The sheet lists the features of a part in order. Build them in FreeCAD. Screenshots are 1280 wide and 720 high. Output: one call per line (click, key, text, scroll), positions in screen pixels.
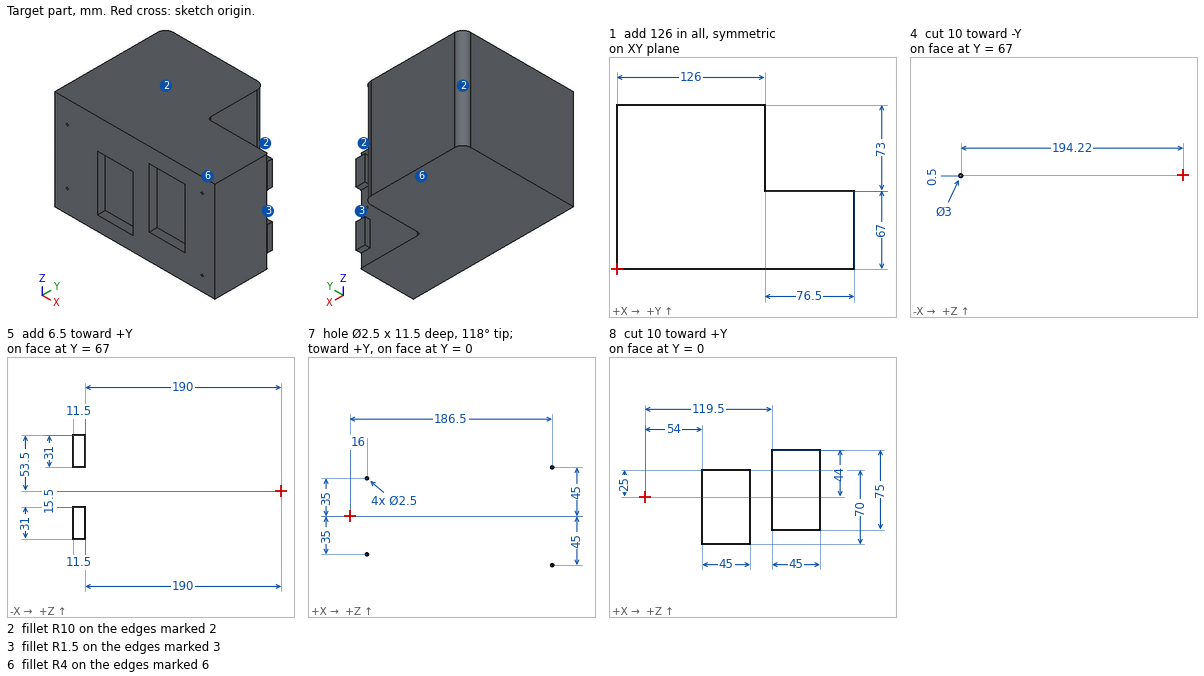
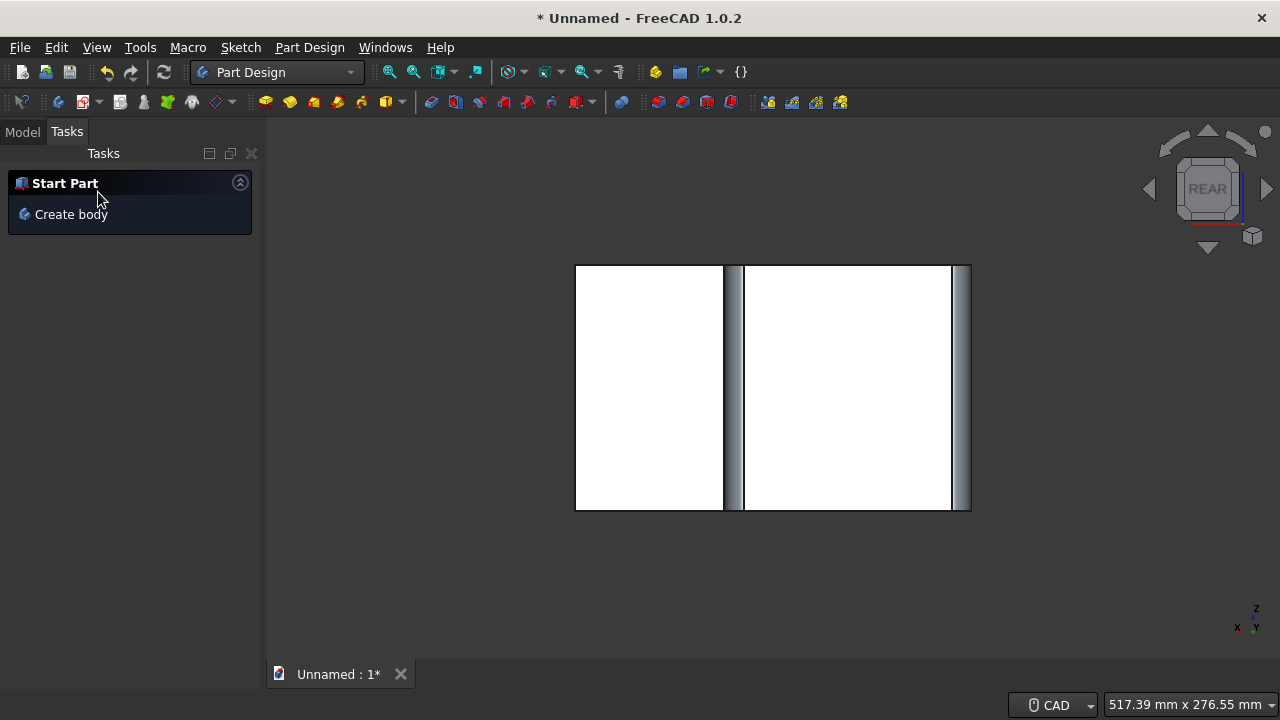
click(575, 387)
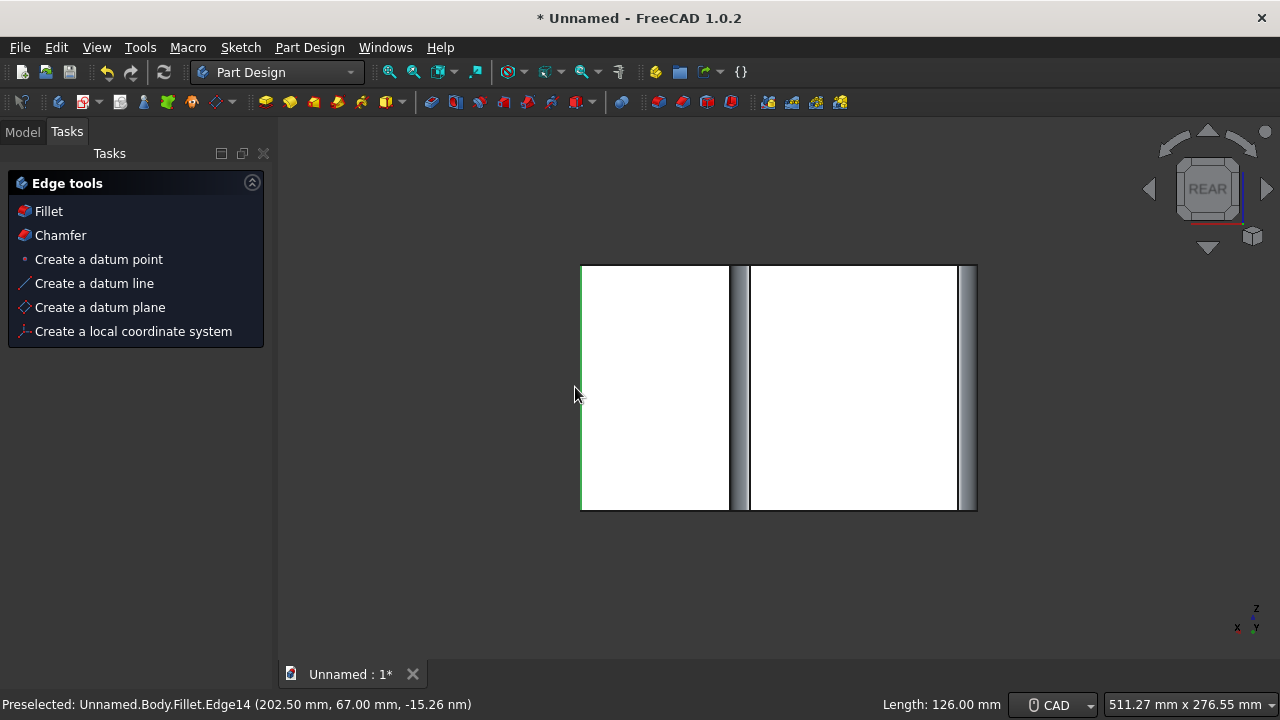
click(660, 102)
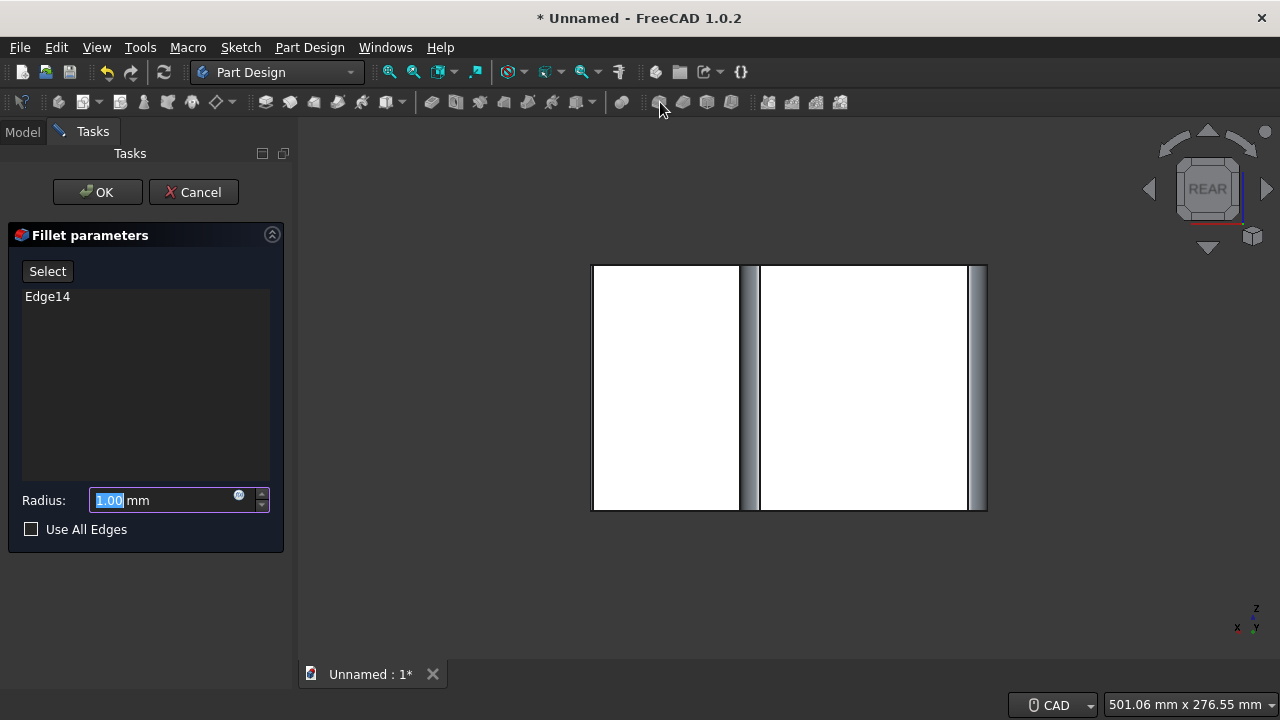
text(1.5)
key(Tab)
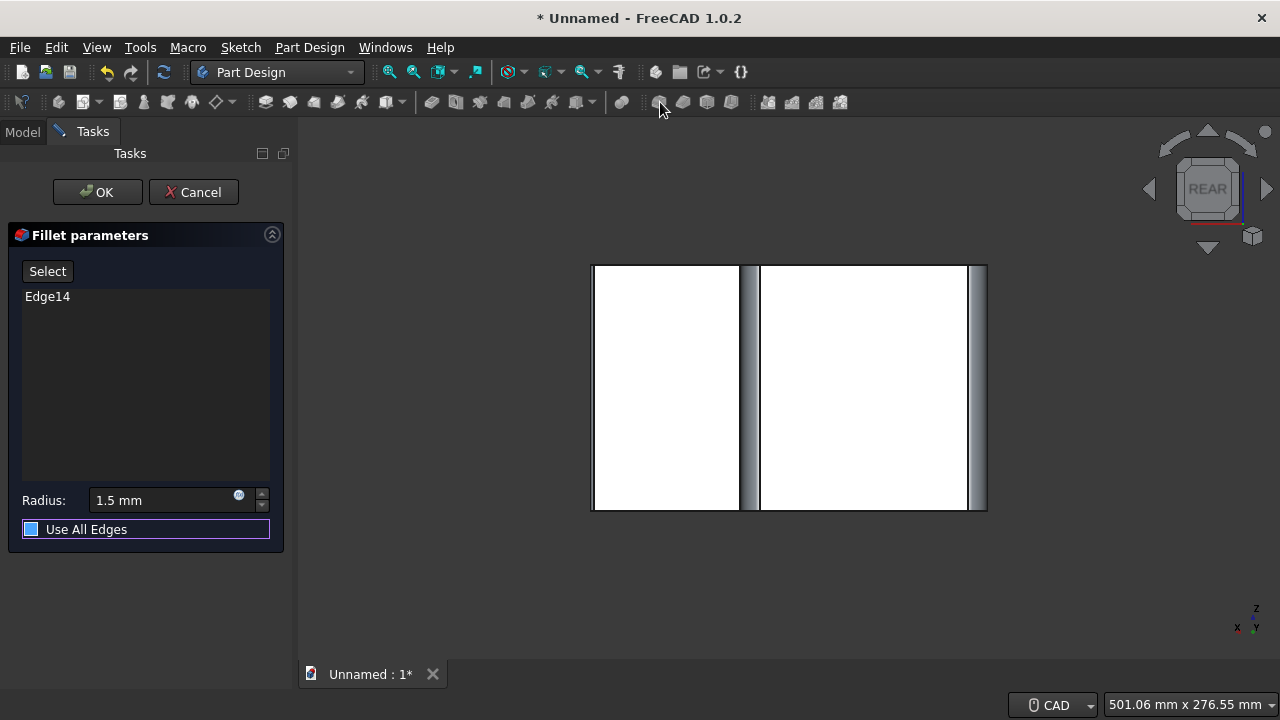
click(98, 192)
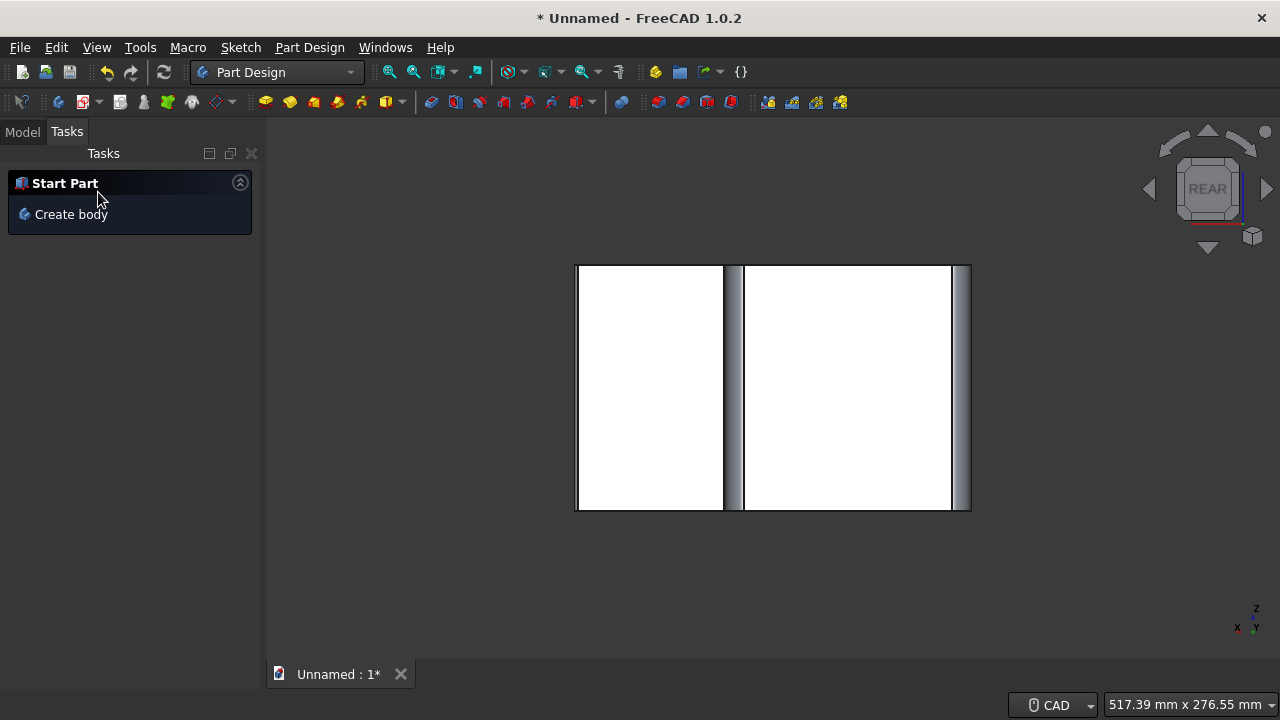
click(651, 352)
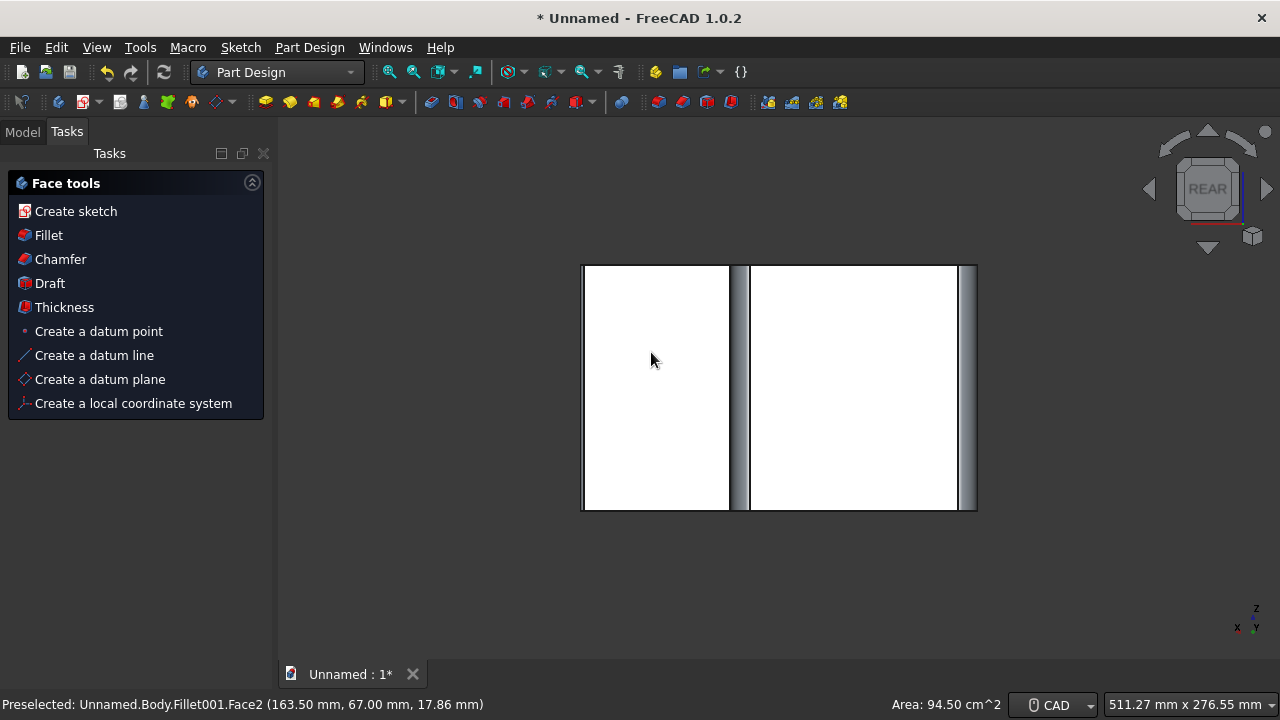
click(84, 102)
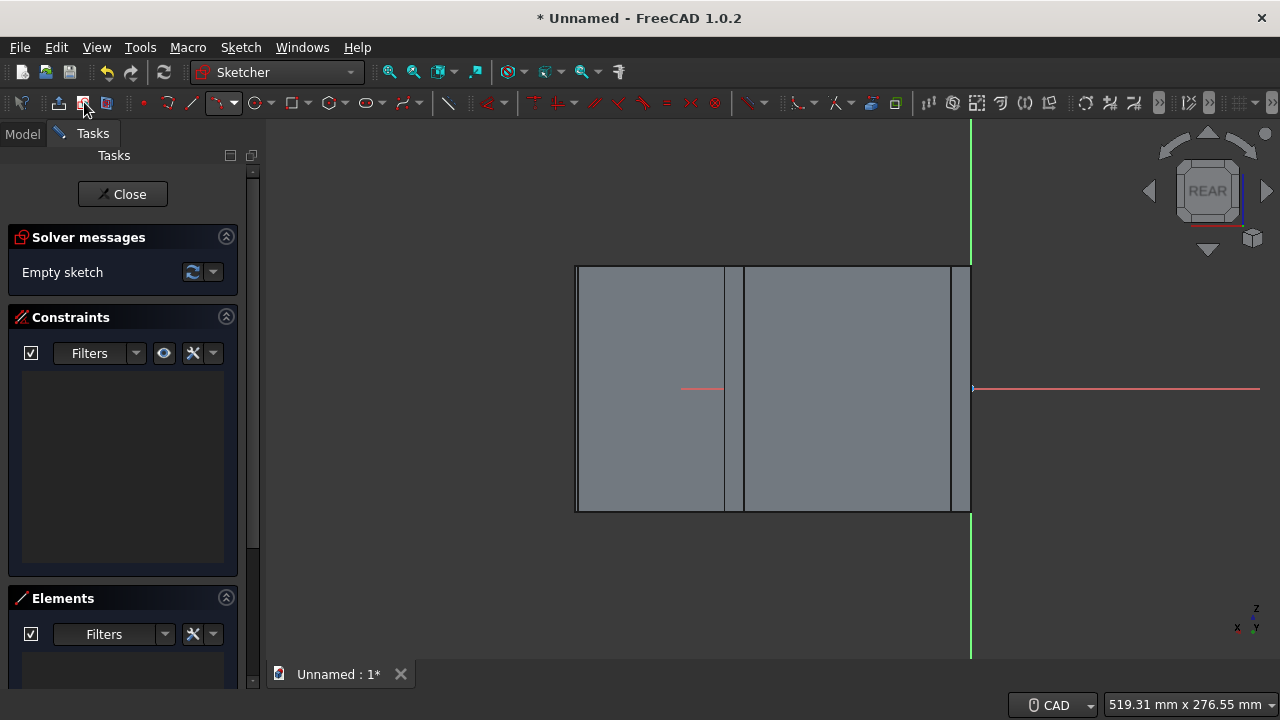
click(108, 104)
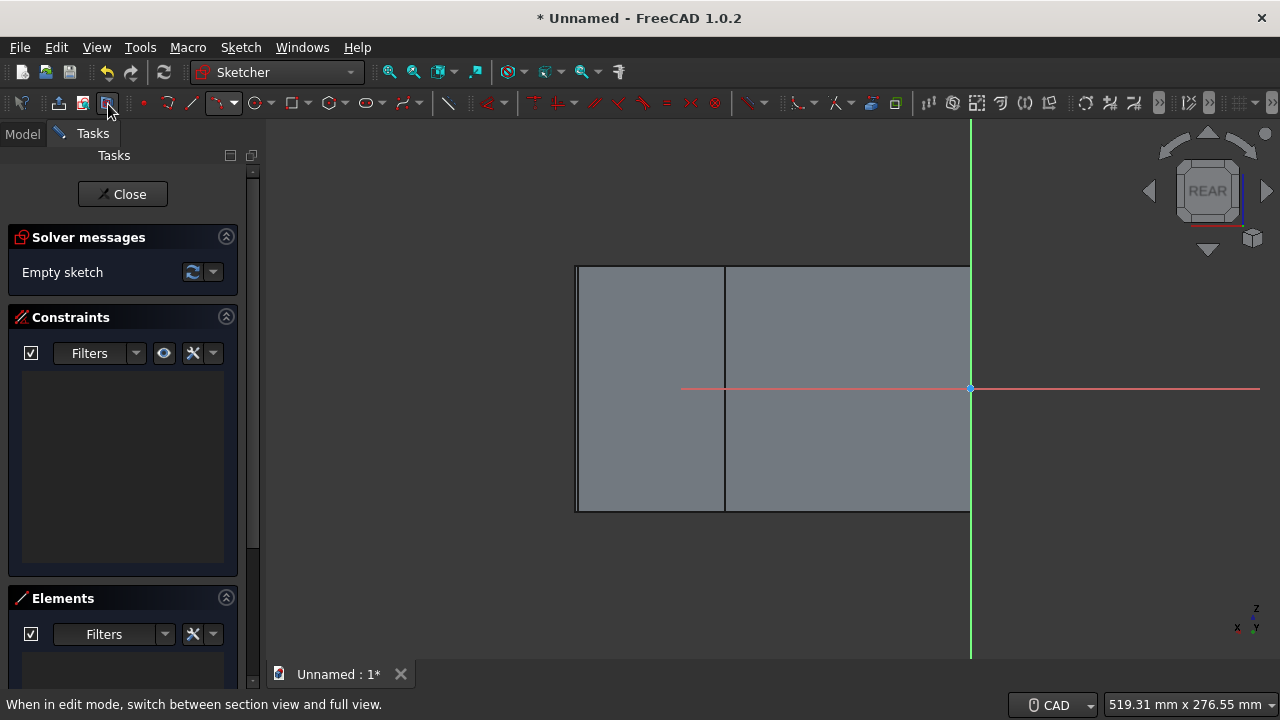
scroll(586, 390, up, 15)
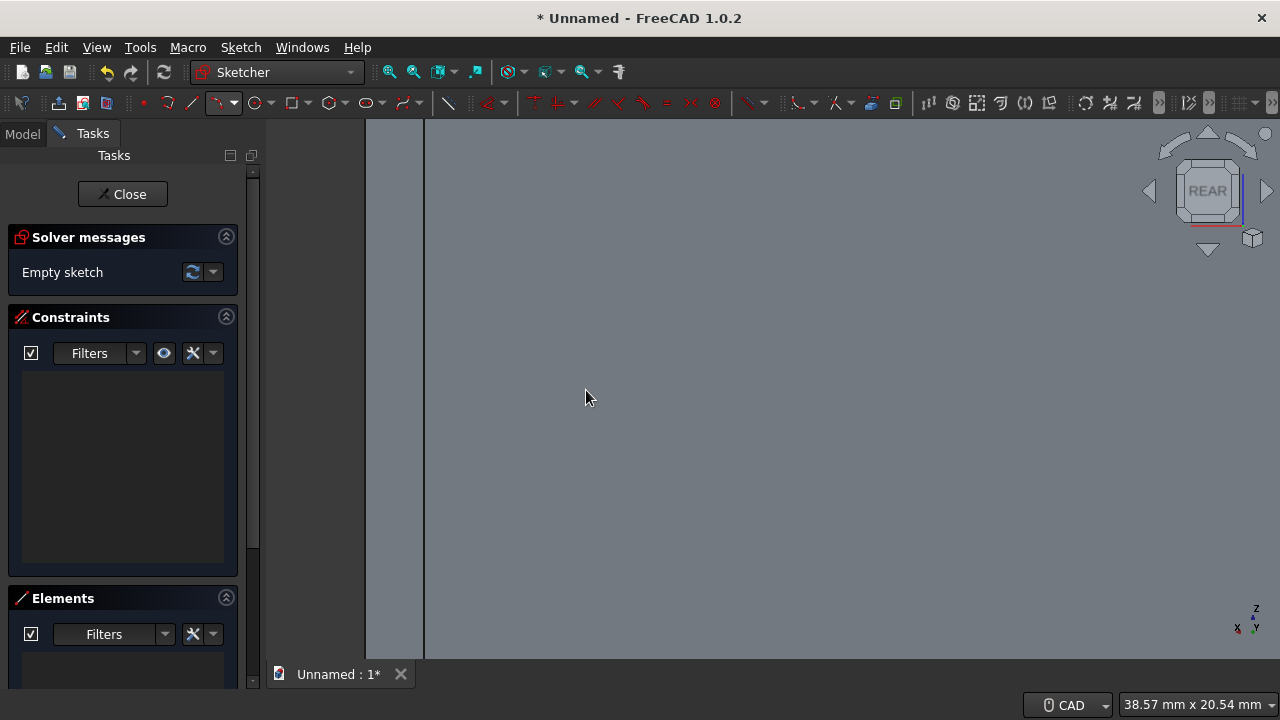
scroll(681, 375, up, 5)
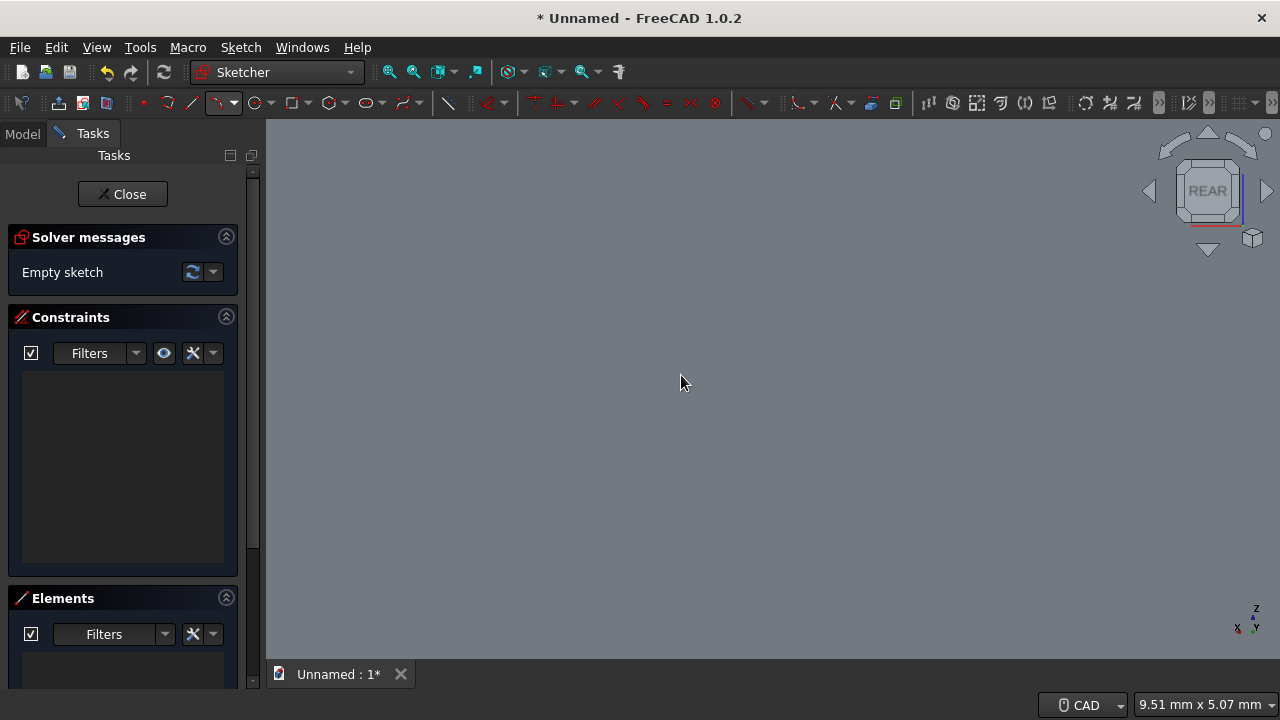
key(g)
key(c)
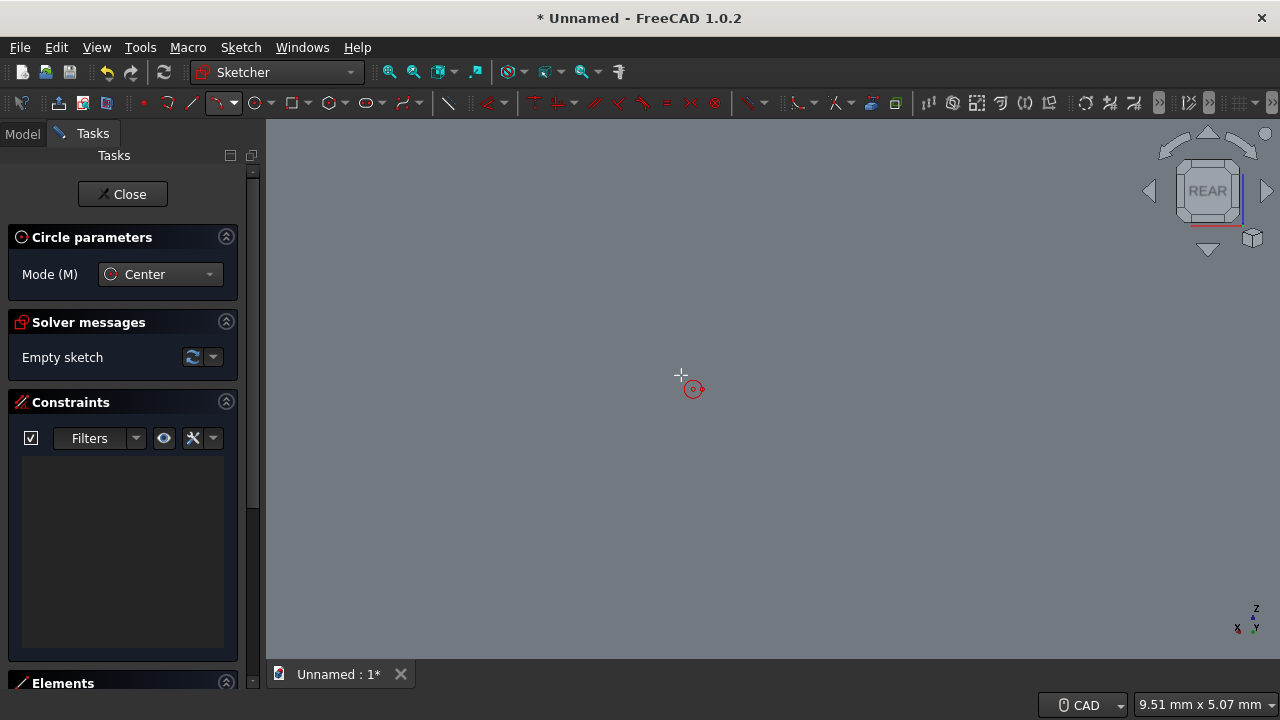
click(704, 388)
move(817, 275)